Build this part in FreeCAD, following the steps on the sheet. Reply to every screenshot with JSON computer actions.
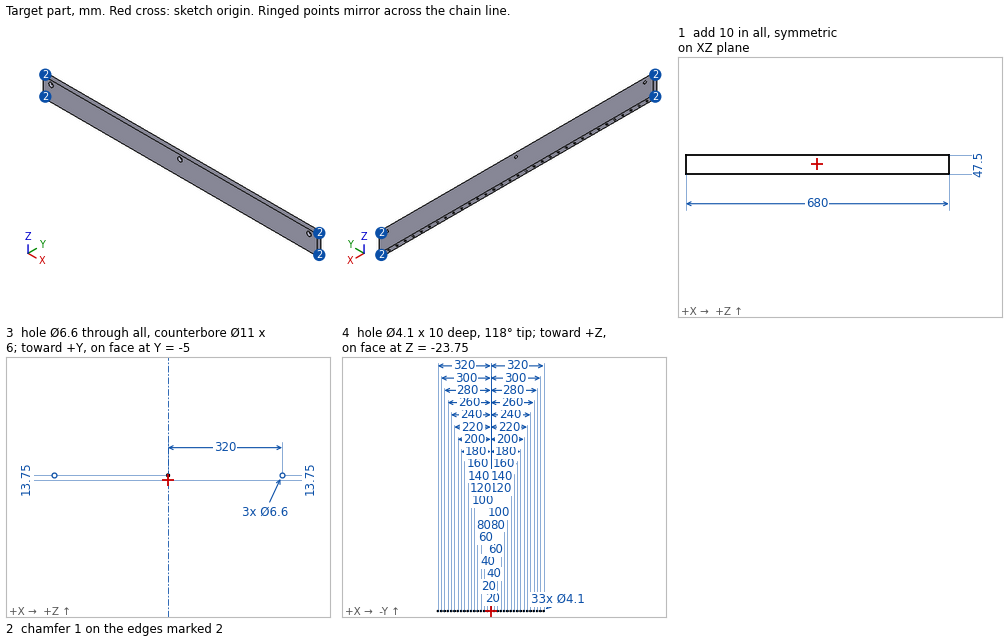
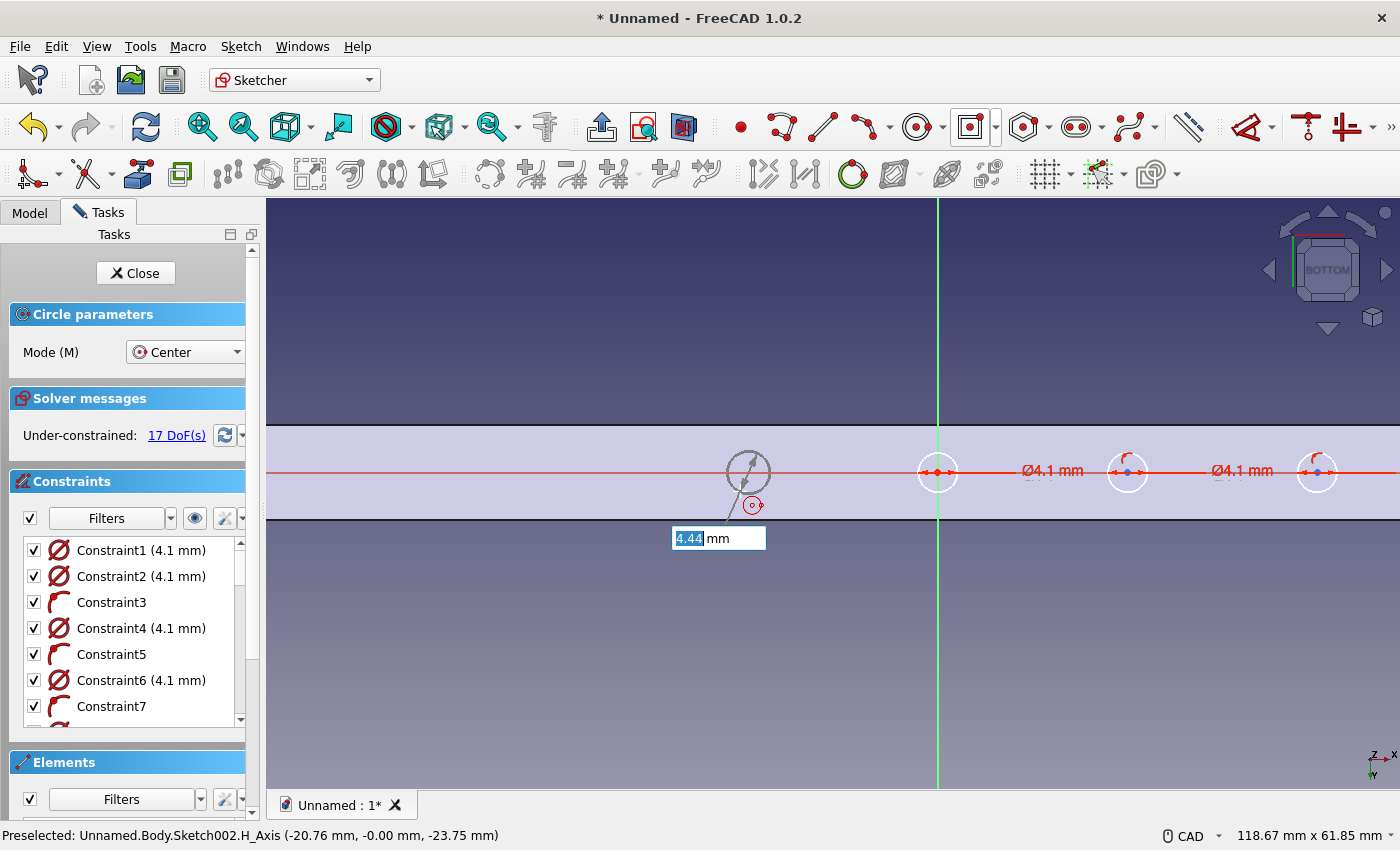
{"action": "type", "text": "4.1"}
{"action": "key", "text": "Return"}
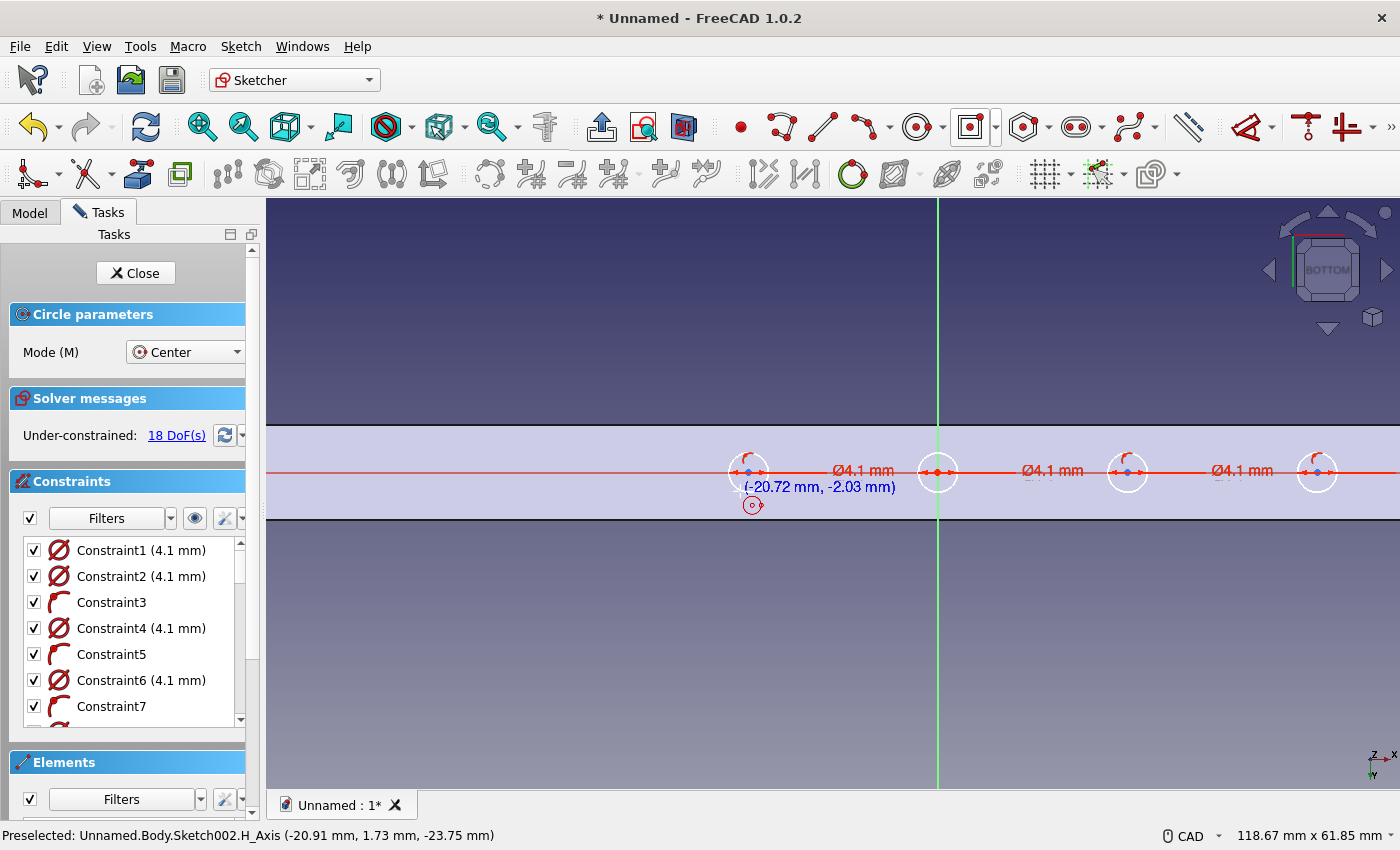
{"action": "scroll", "coordinate": [743, 496], "scroll_direction": "down", "scroll_amount": 11}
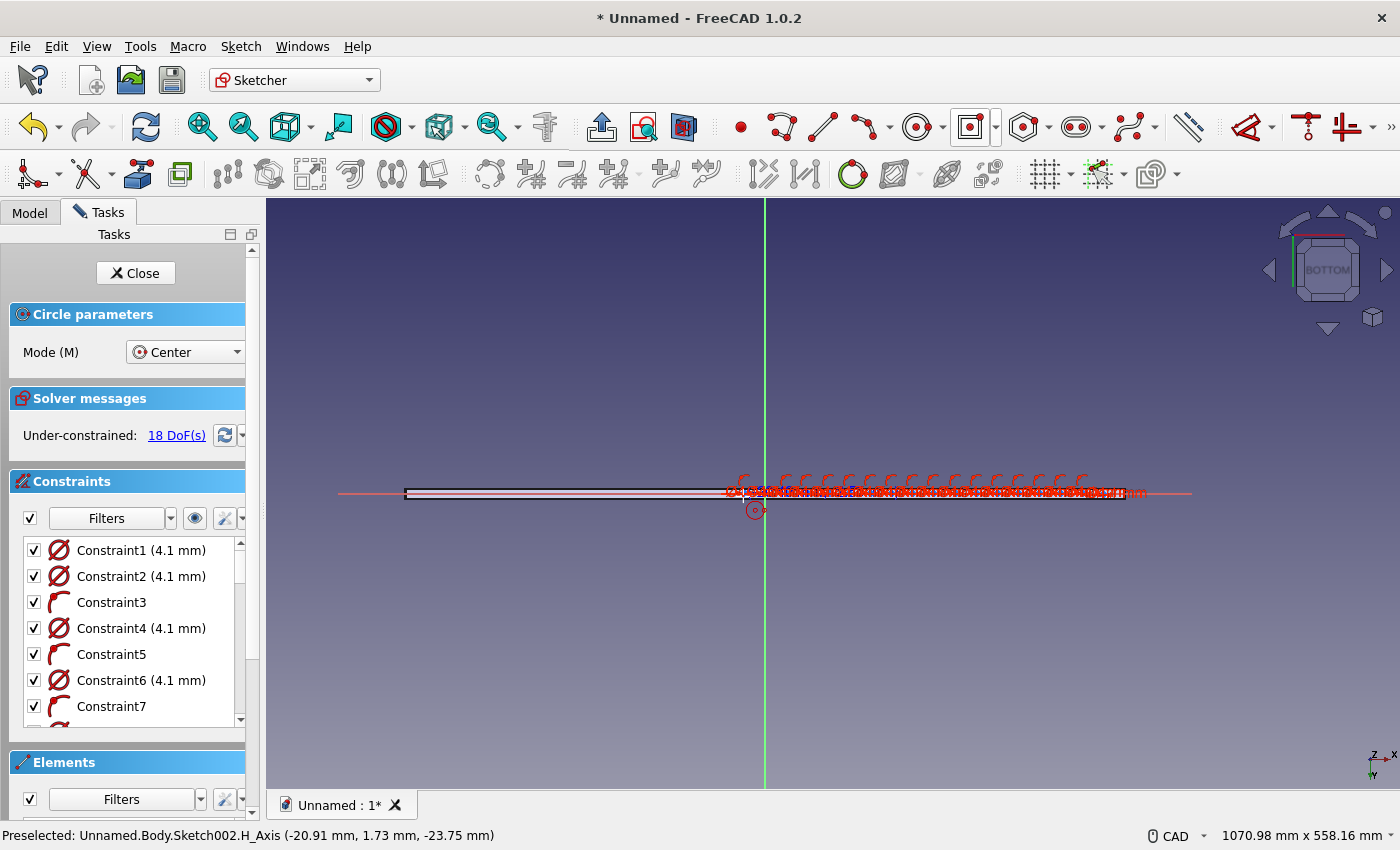
{"action": "left_click", "coordinate": [723, 494]}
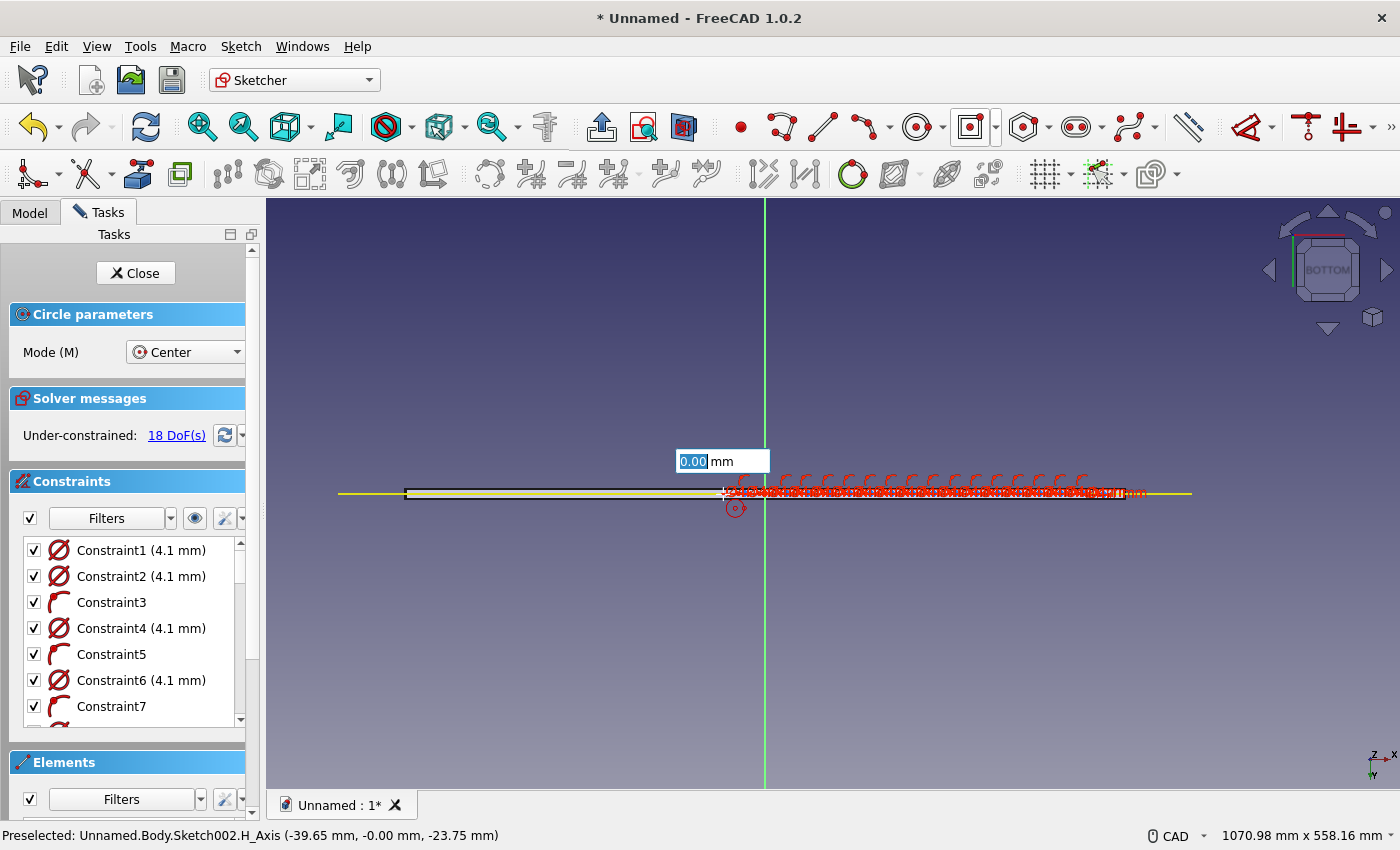
{"action": "scroll", "coordinate": [723, 492], "scroll_direction": "up", "scroll_amount": 11}
{"action": "mouse_move", "coordinate": [723, 486]}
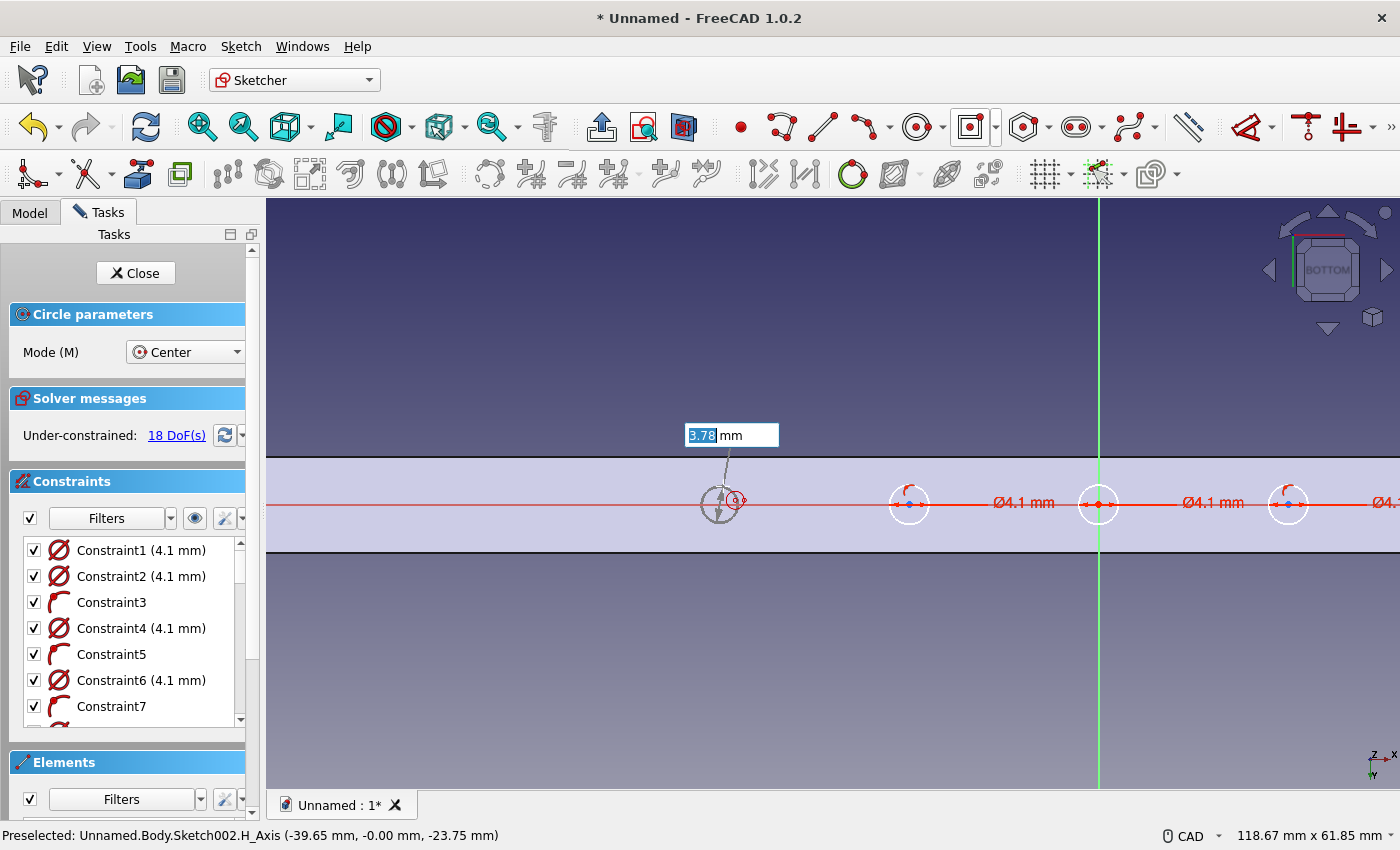
{"action": "type", "text": "4.1"}
{"action": "key", "text": "Return"}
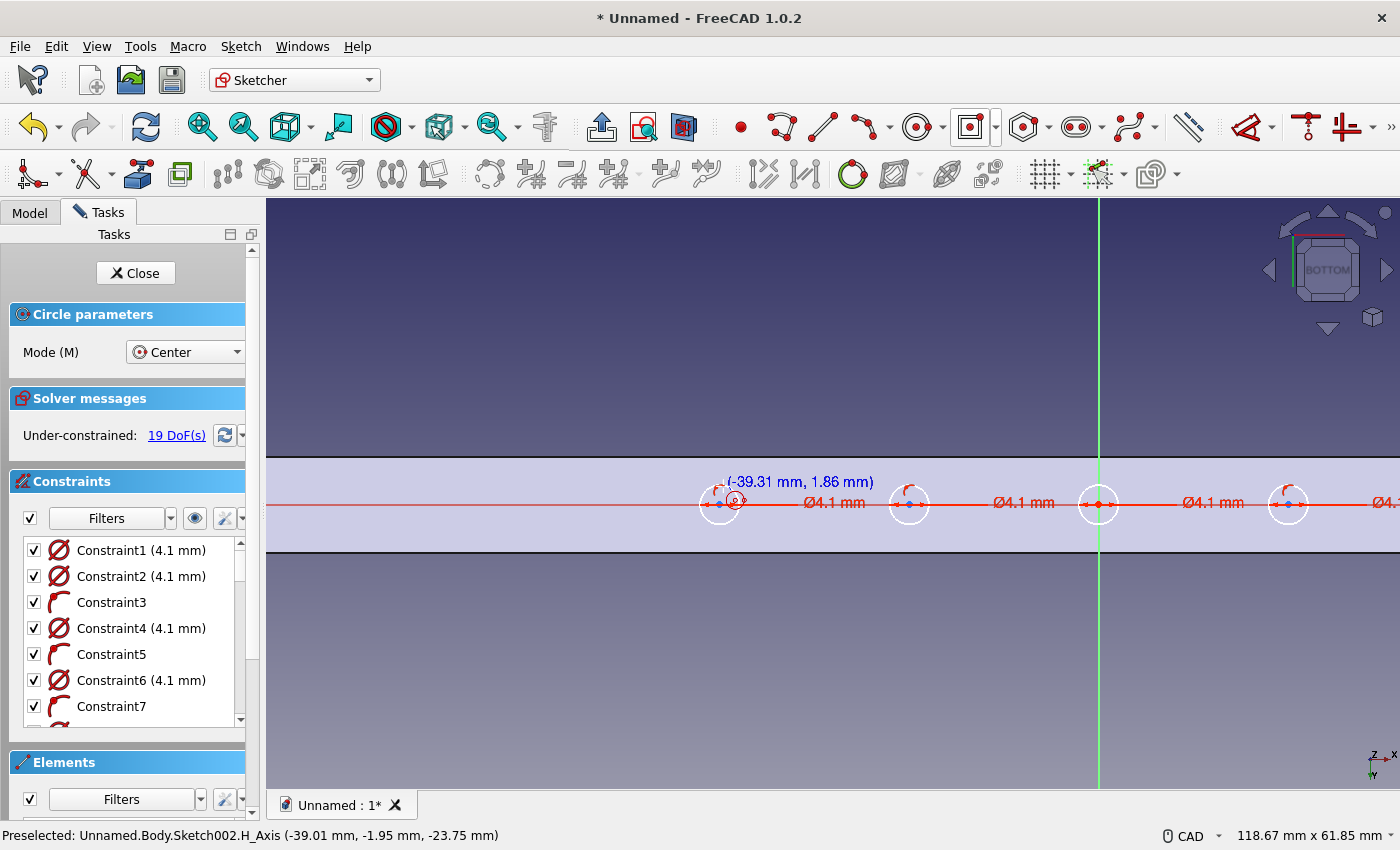
{"action": "scroll", "coordinate": [723, 492], "scroll_direction": "down", "scroll_amount": 11}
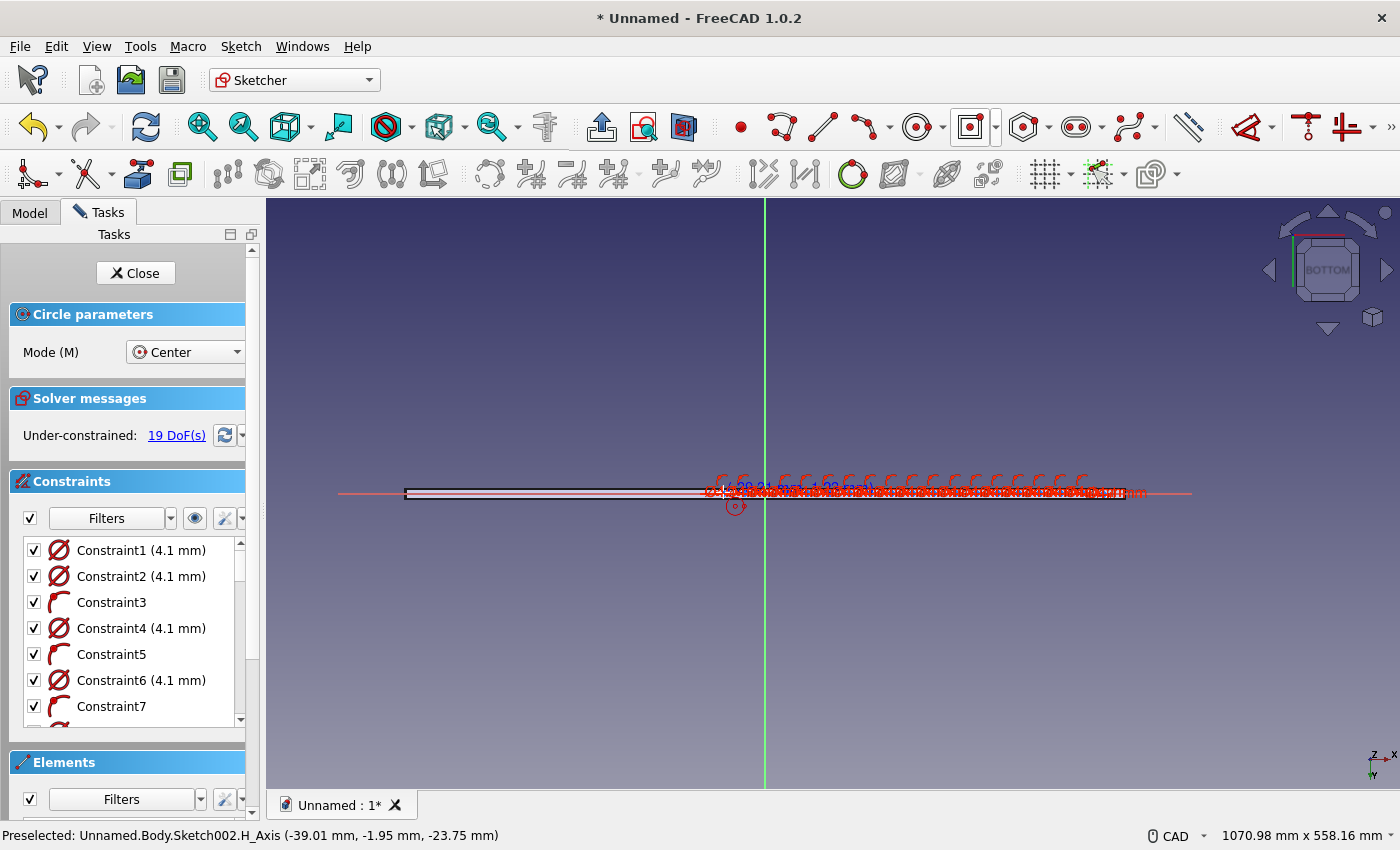
{"action": "left_click", "coordinate": [701, 494]}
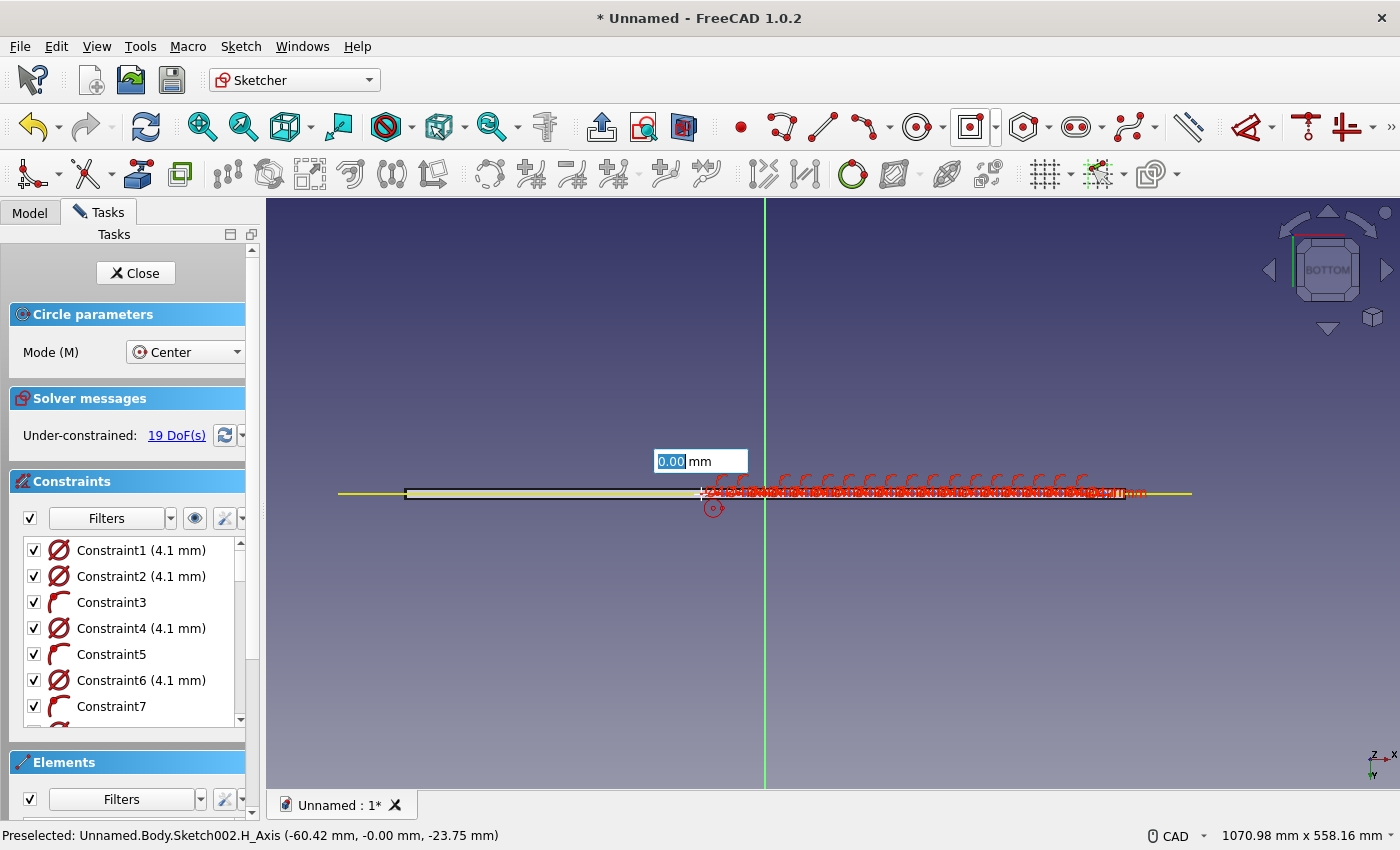
{"action": "scroll", "coordinate": [701, 496], "scroll_direction": "up", "scroll_amount": 11}
{"action": "mouse_move", "coordinate": [695, 491]}